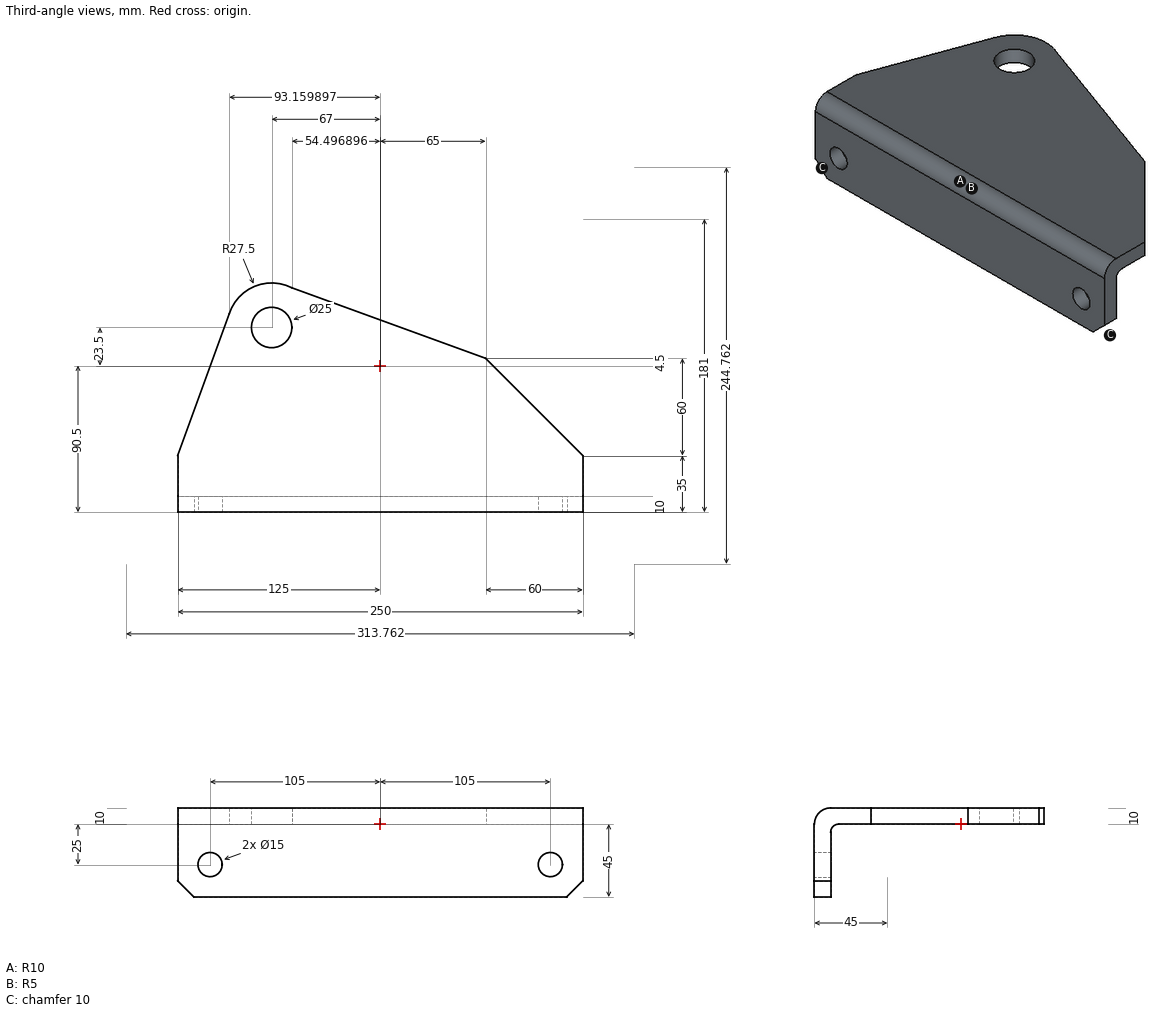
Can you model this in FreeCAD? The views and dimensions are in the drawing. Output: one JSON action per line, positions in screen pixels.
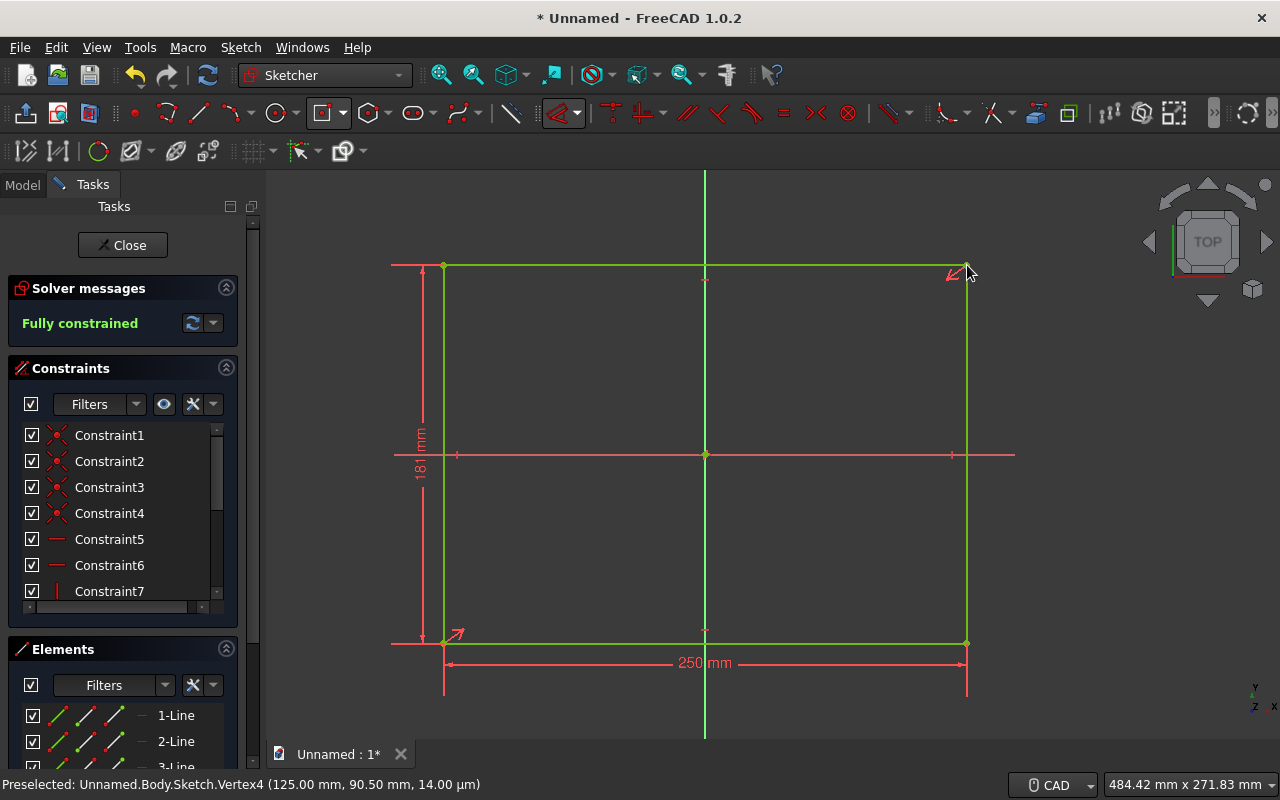
{"action": "left_click", "coordinate": [123, 245]}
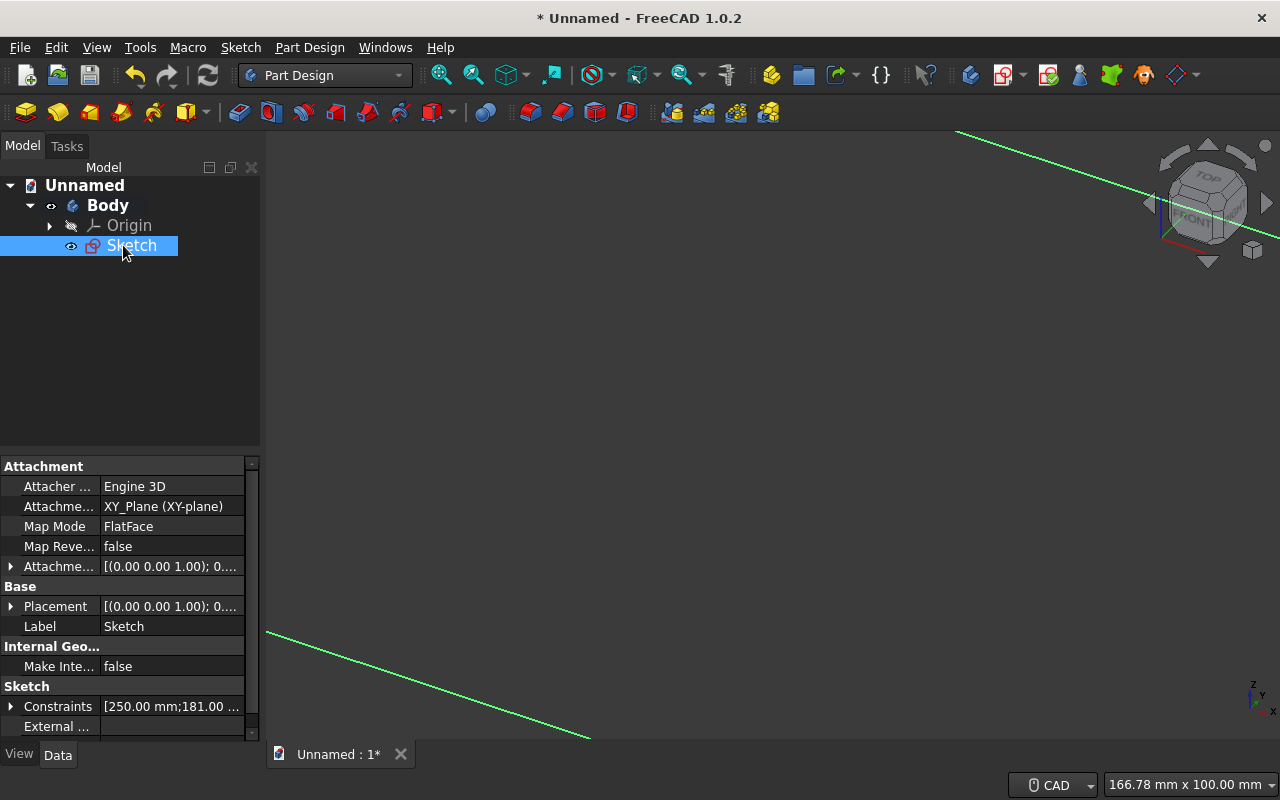
{"action": "left_click", "coordinate": [26, 112]}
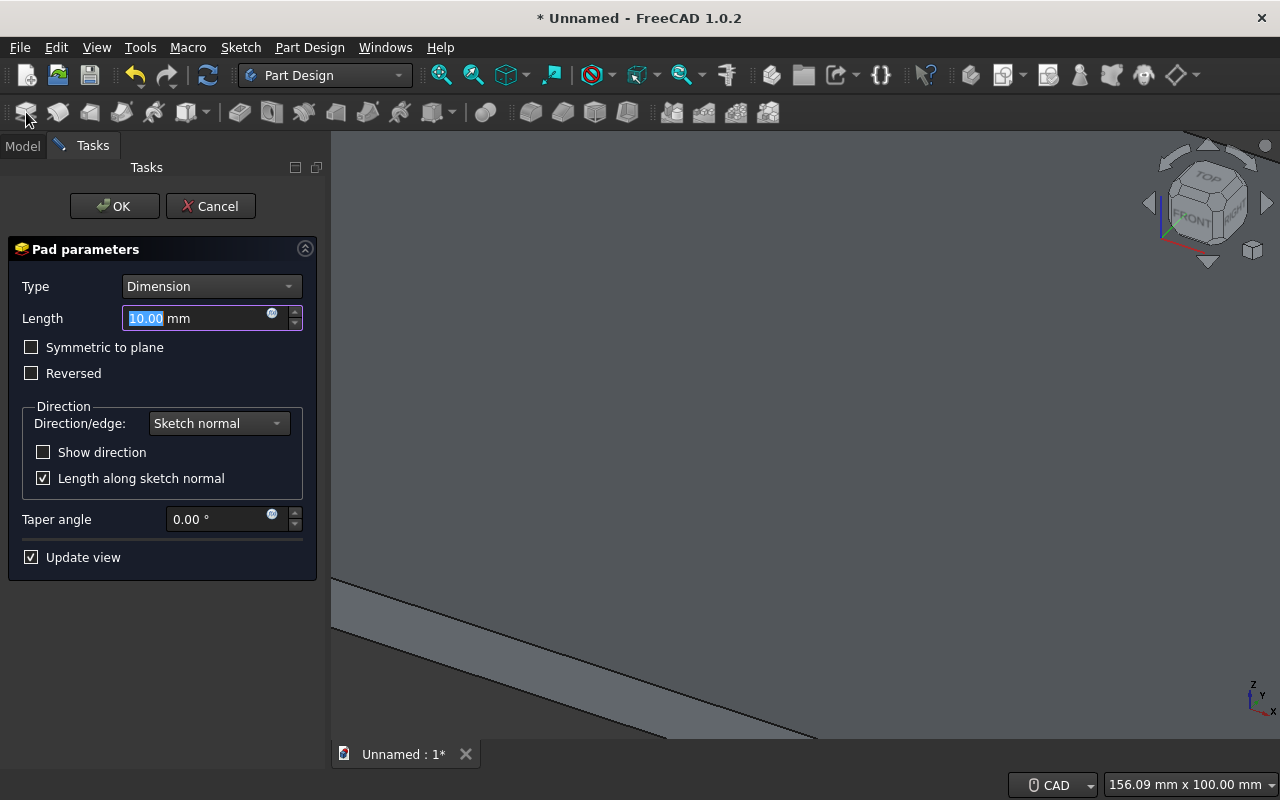
{"action": "type", "text": "10"}
{"action": "key", "text": "Tab"}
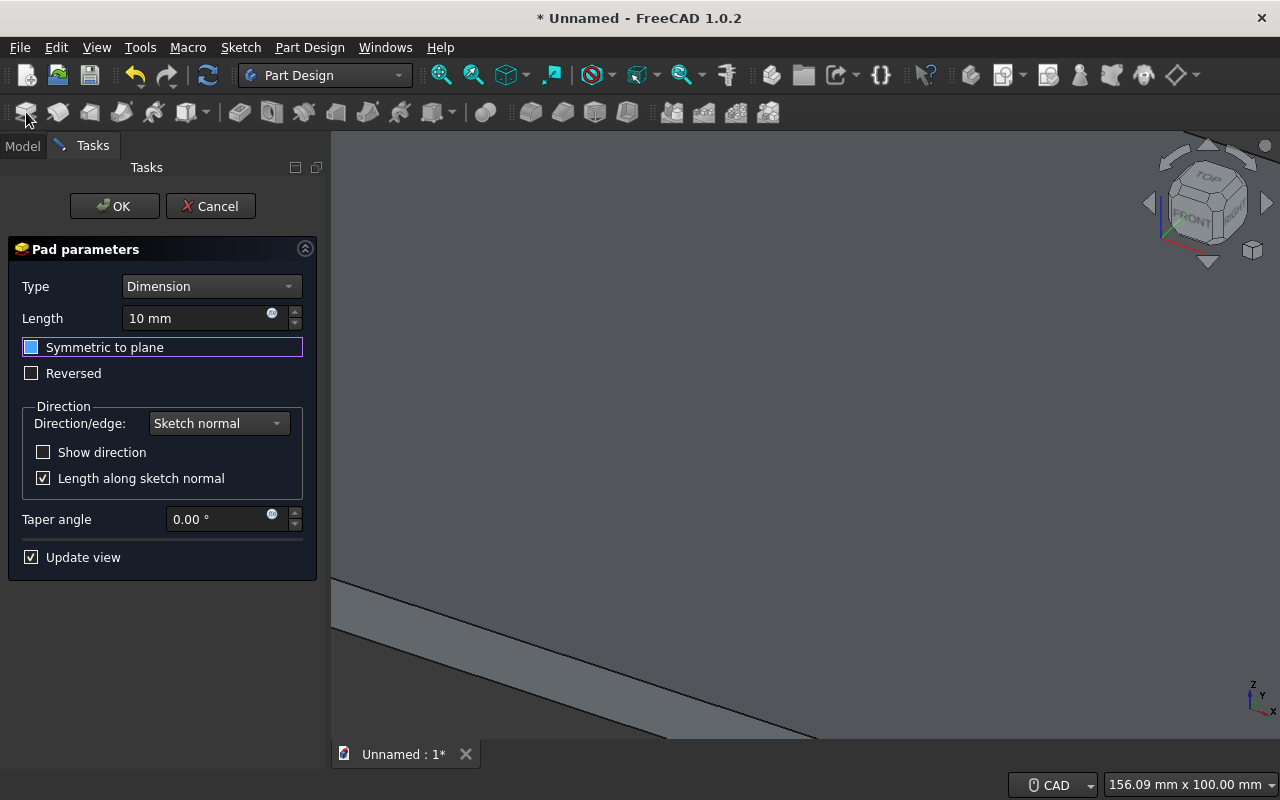
{"action": "left_click", "coordinate": [115, 206]}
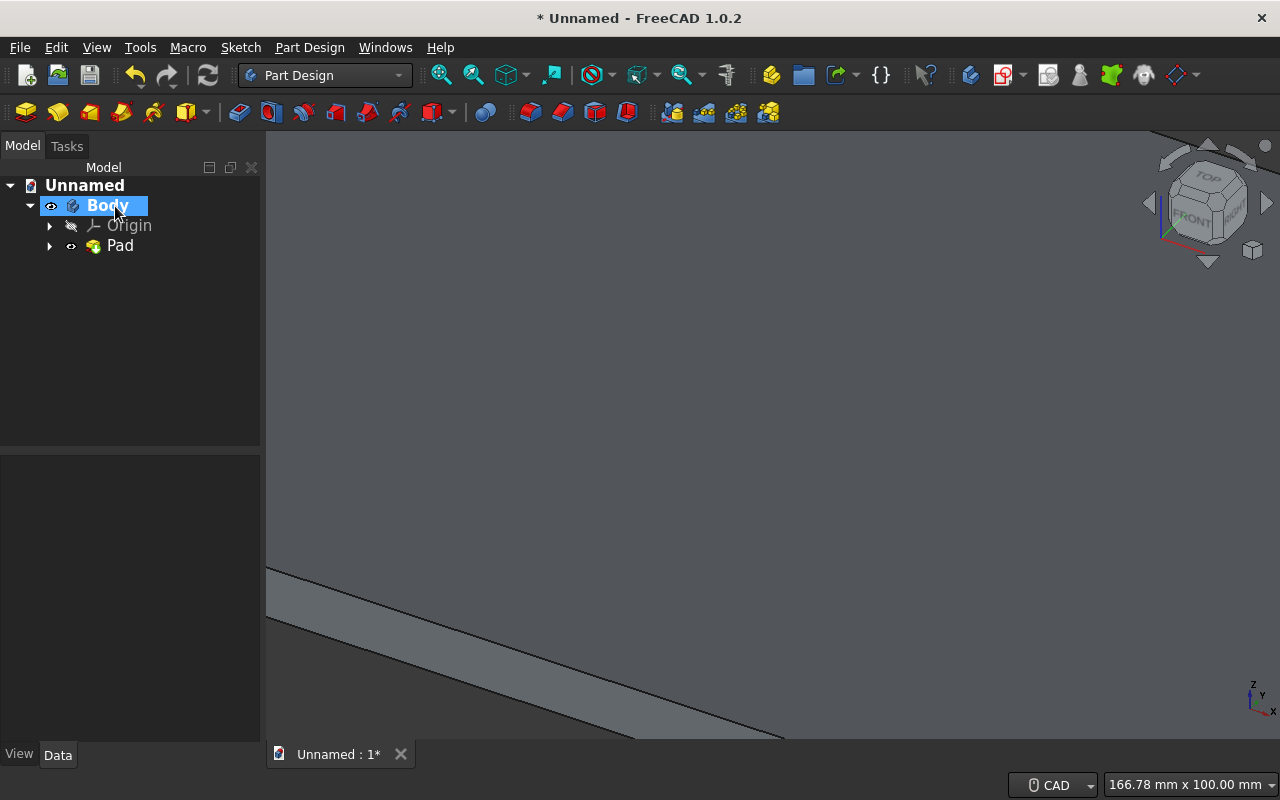
{"action": "left_click", "coordinate": [442, 76]}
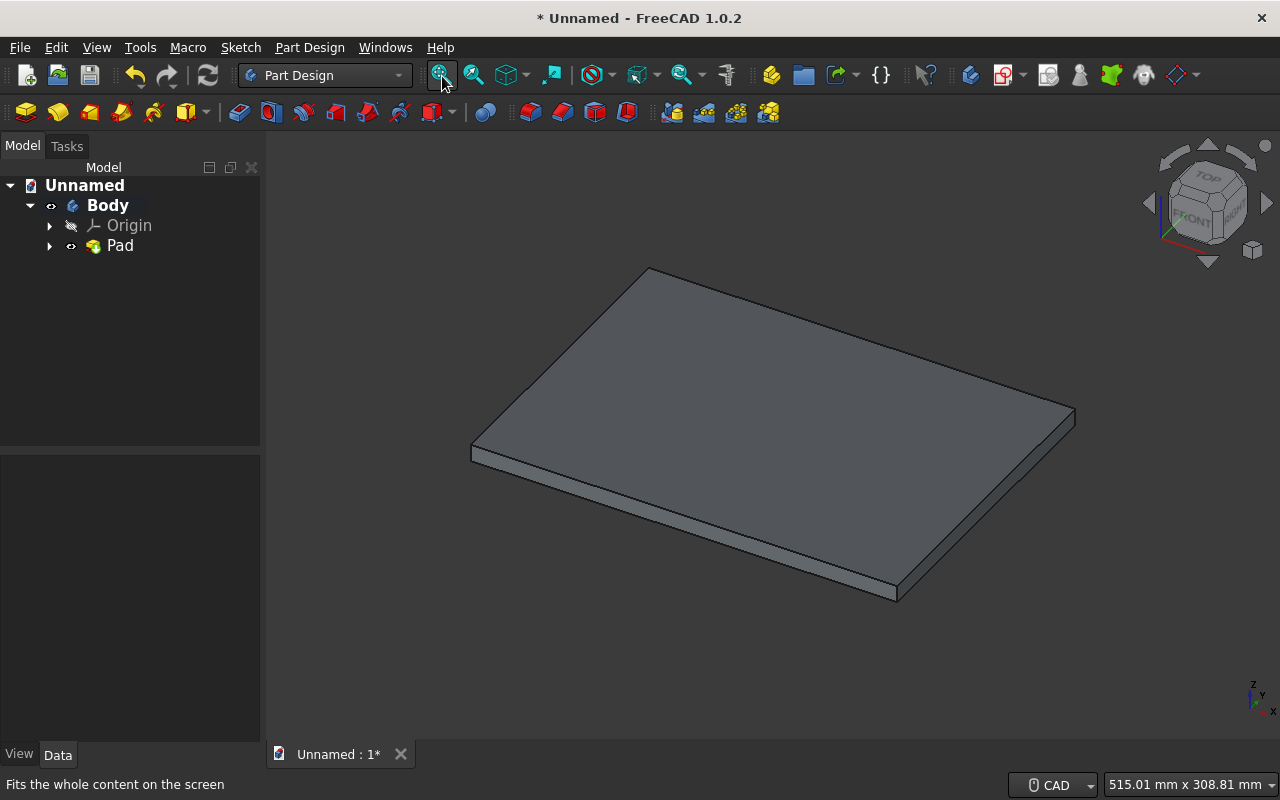
{"action": "left_click", "coordinate": [773, 426]}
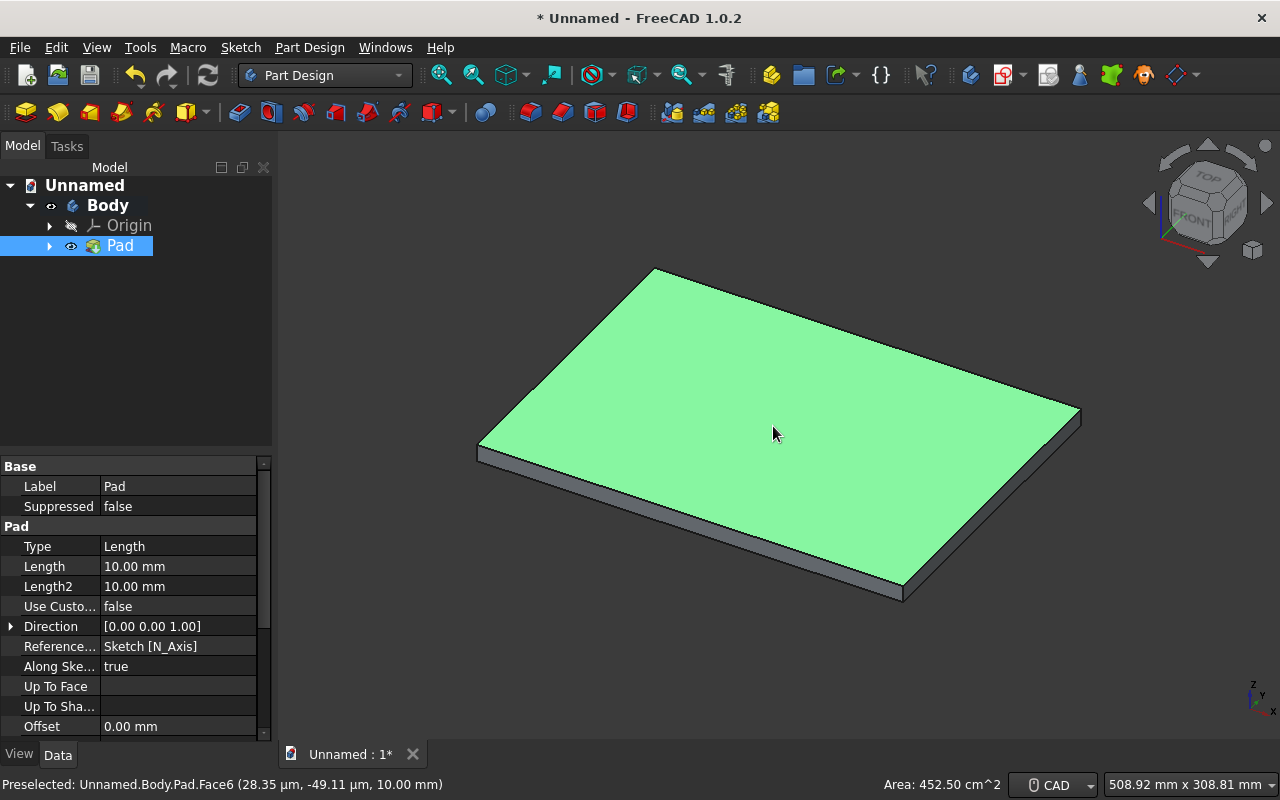
{"action": "left_click", "coordinate": [1004, 76]}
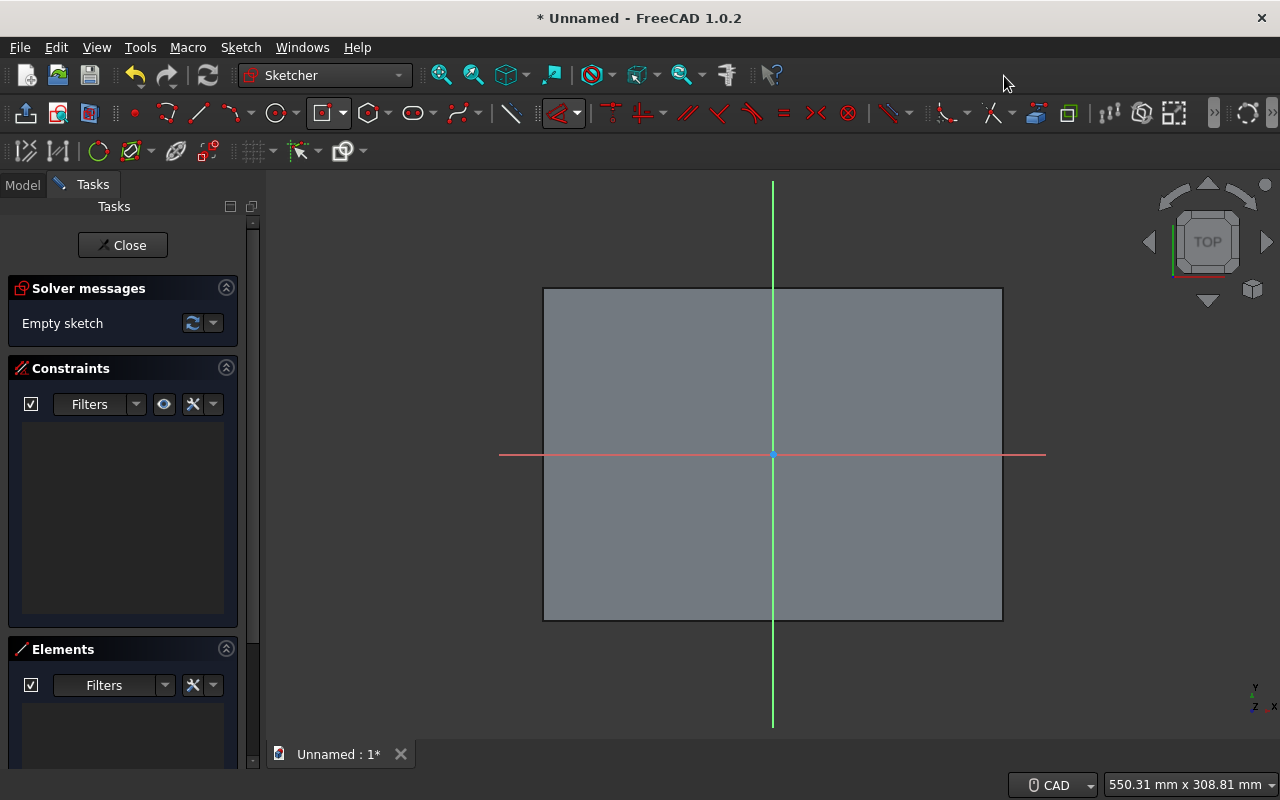
{"action": "key", "text": "g v"}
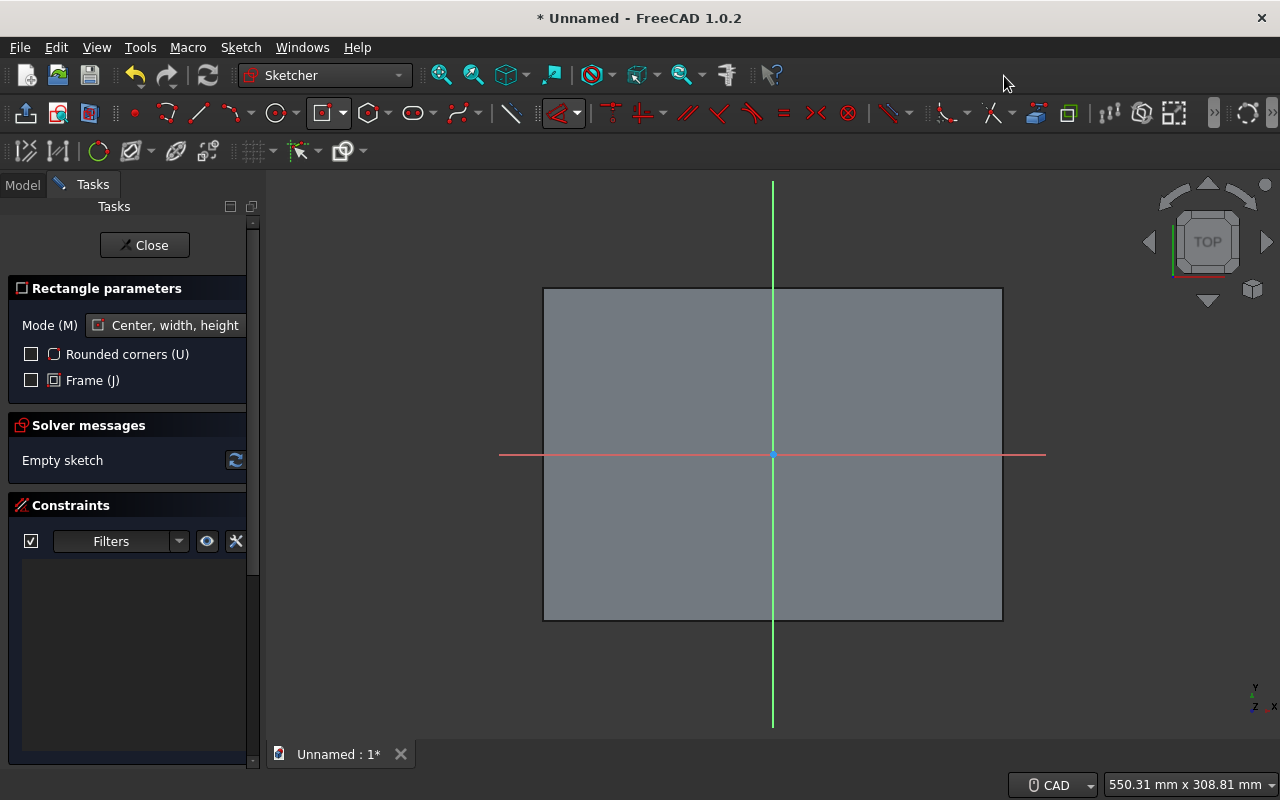
{"action": "left_click", "coordinate": [773, 454]}
{"action": "mouse_move", "coordinate": [1062, 229]}